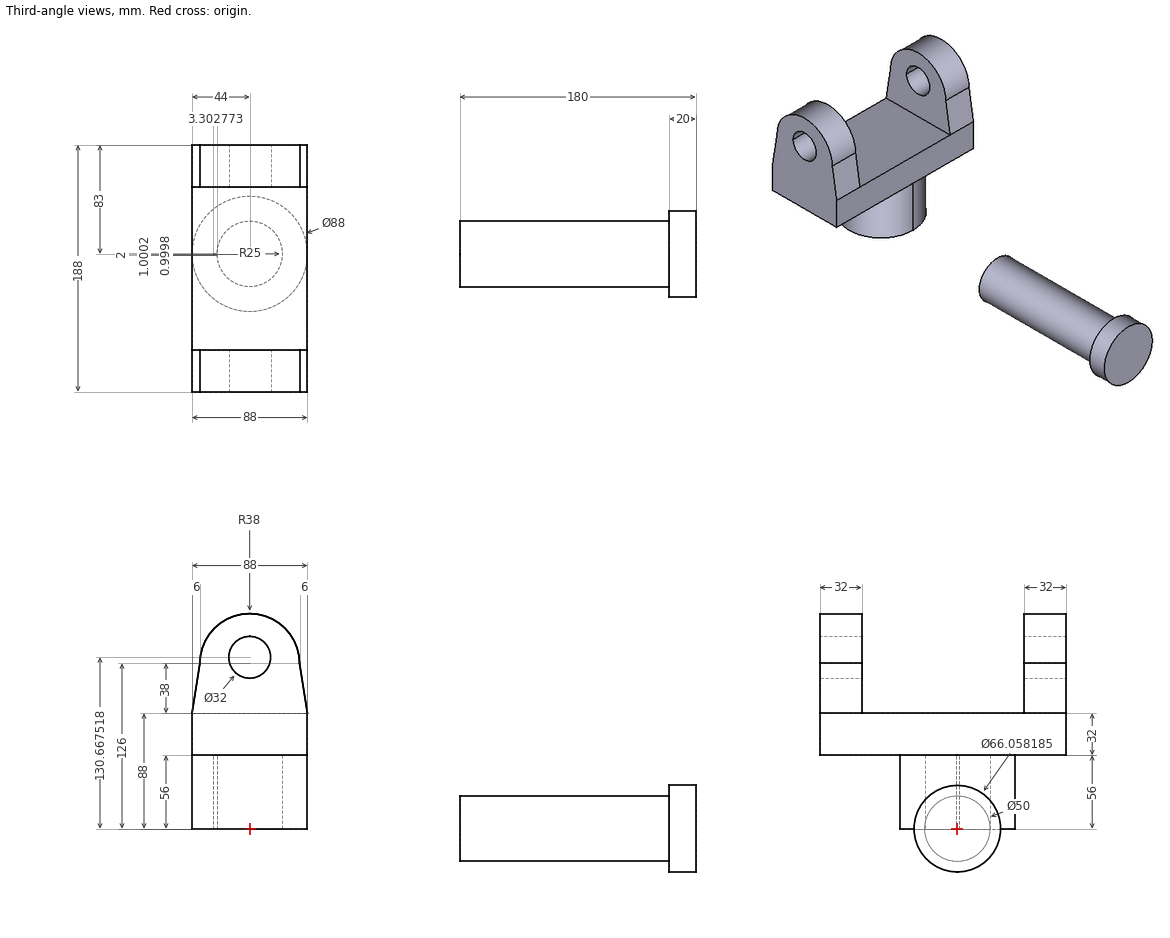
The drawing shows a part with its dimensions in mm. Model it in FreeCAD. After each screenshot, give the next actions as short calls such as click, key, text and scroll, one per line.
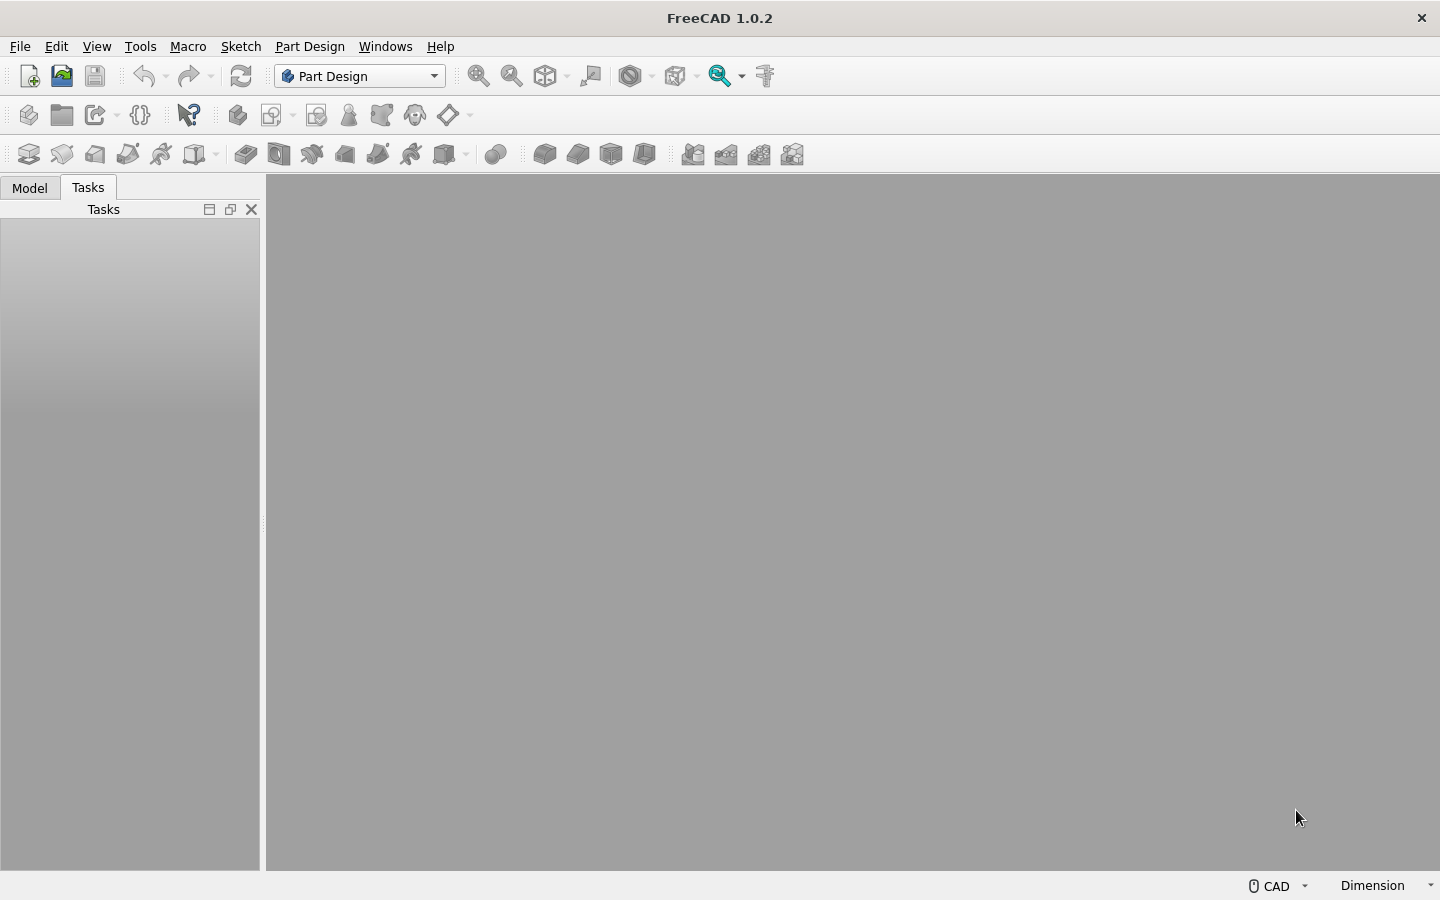
key(ctrl+n)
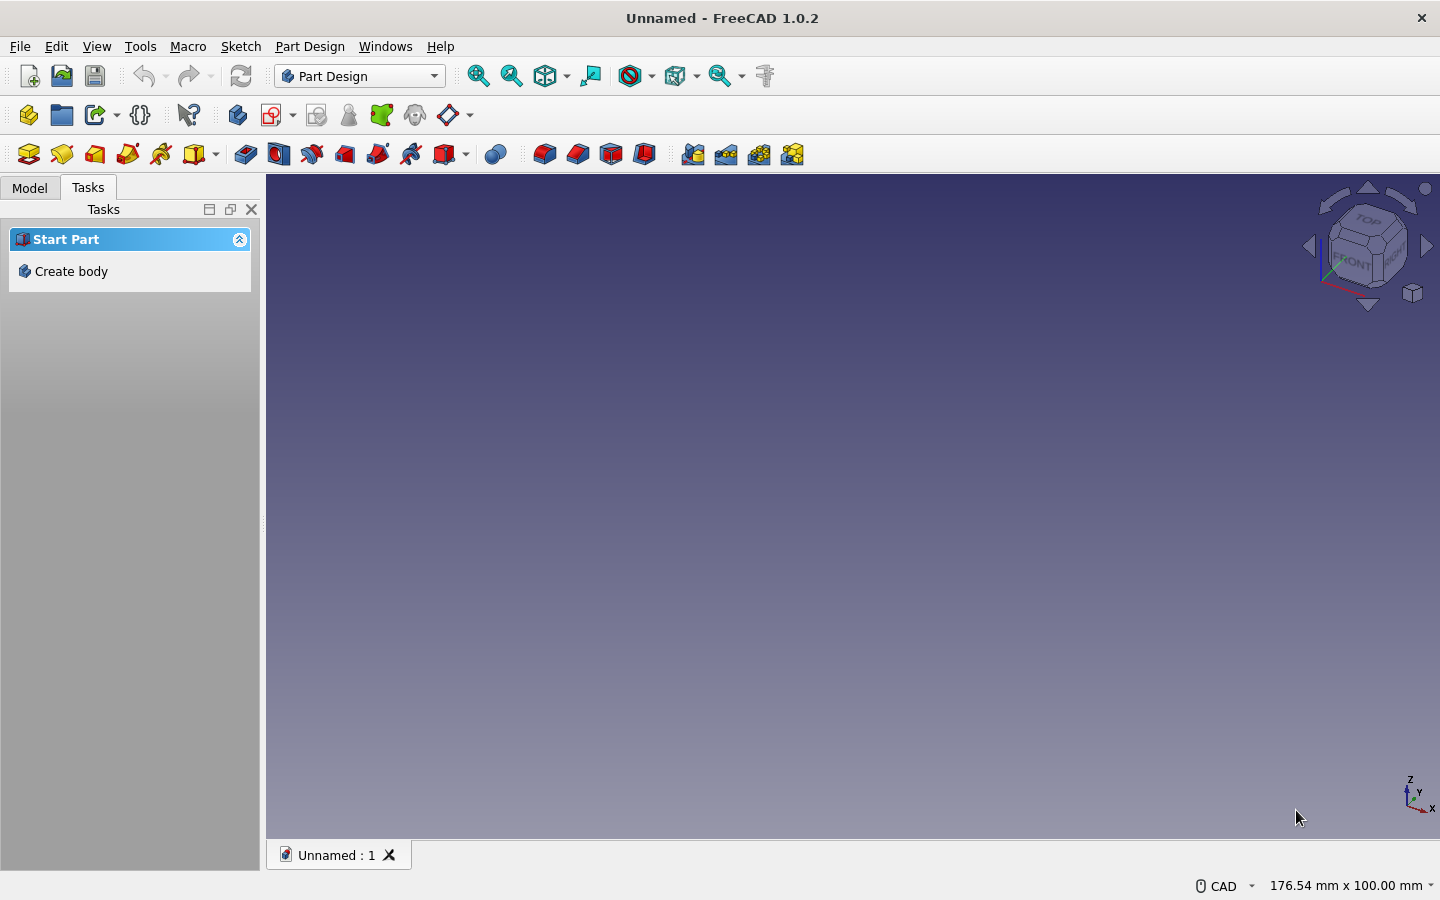
click(270, 116)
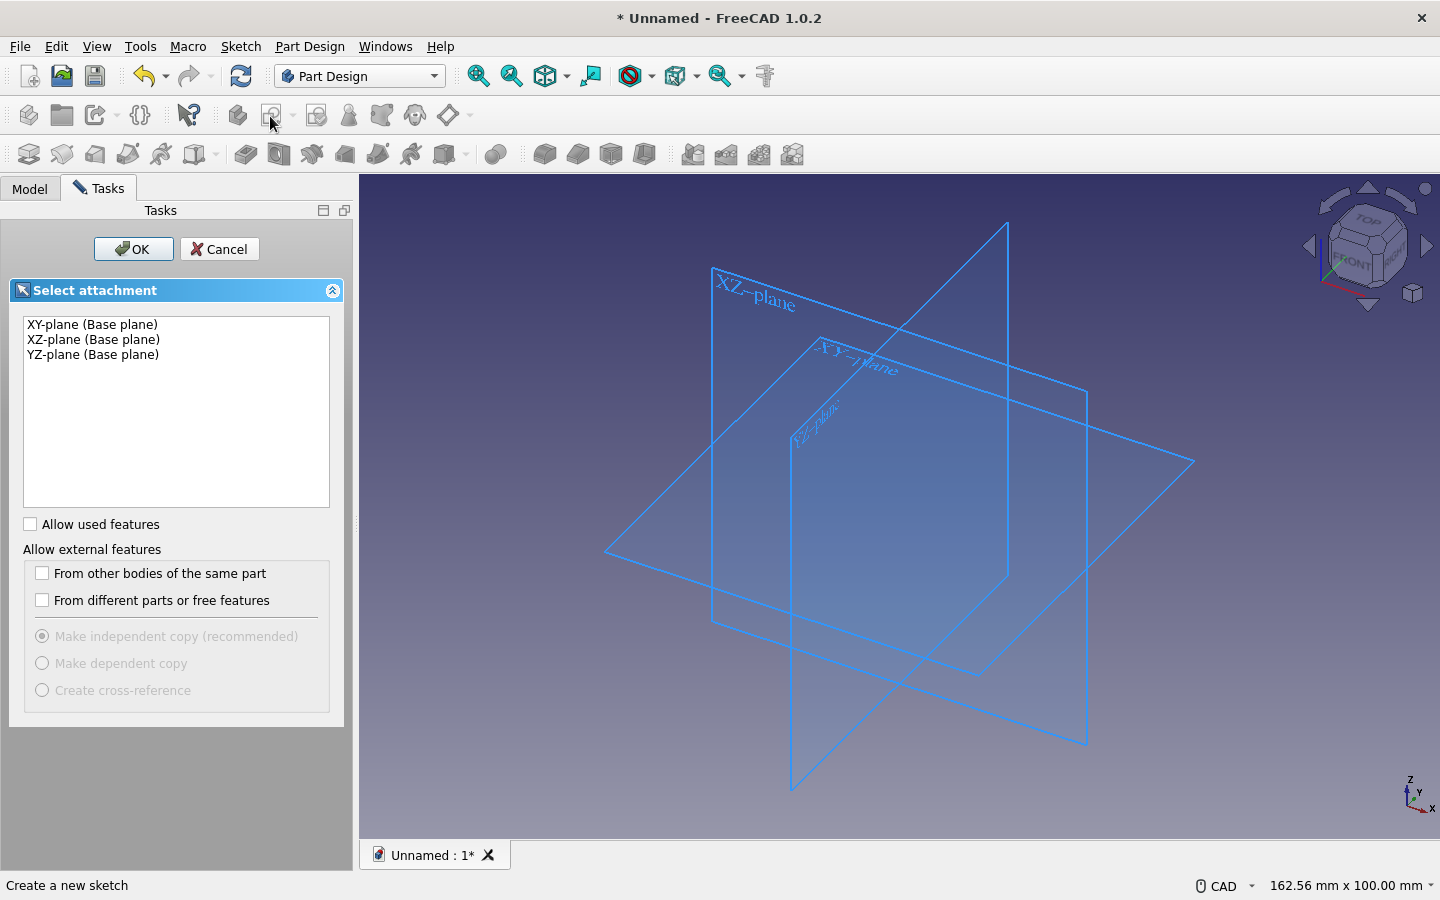
click(84, 324)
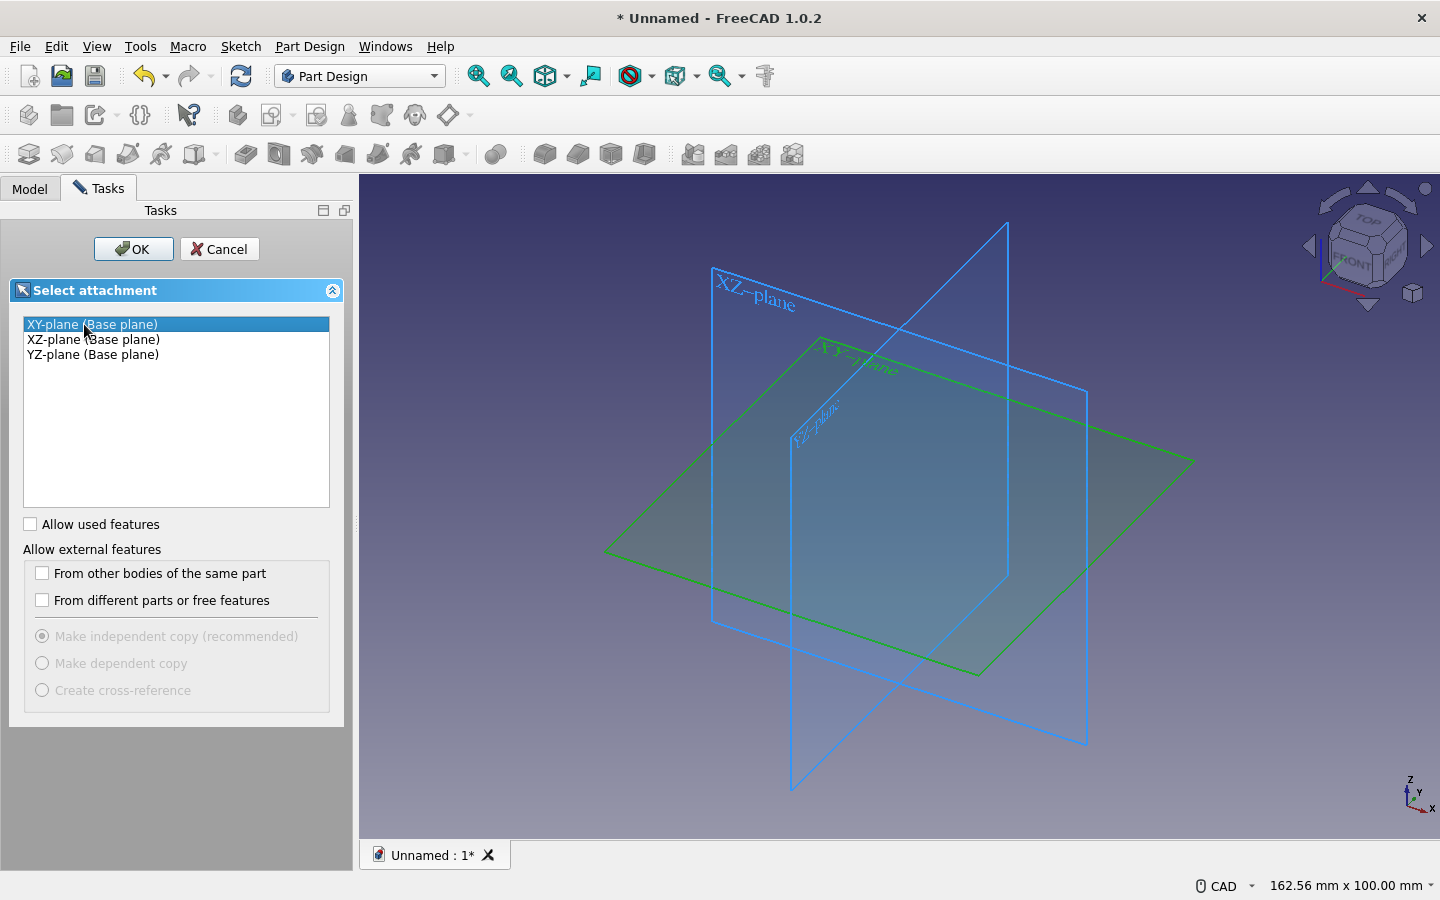
click(134, 249)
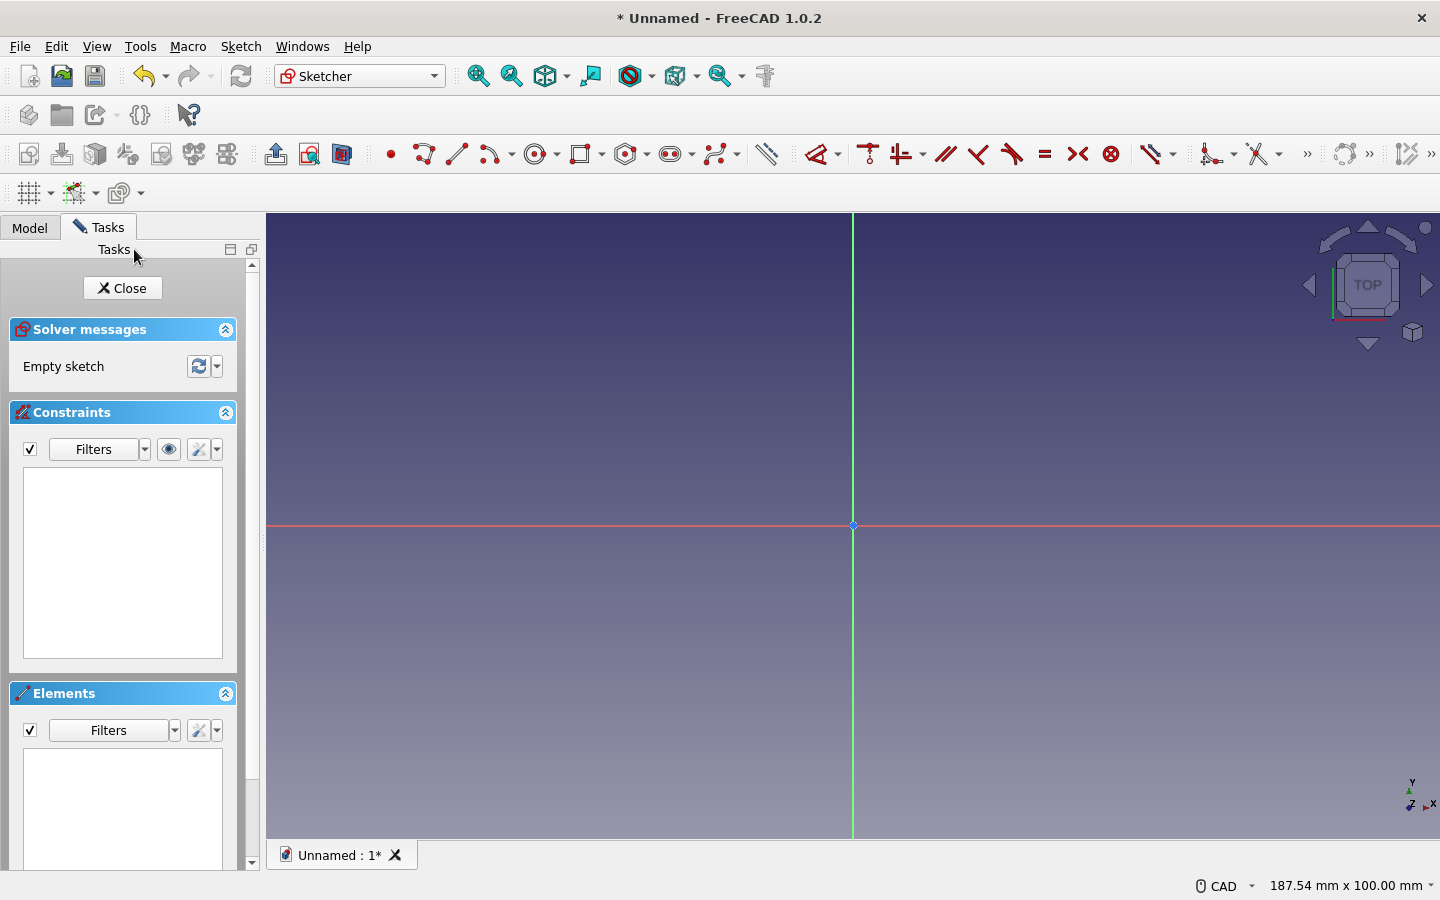
scroll(645, 526, down, 2)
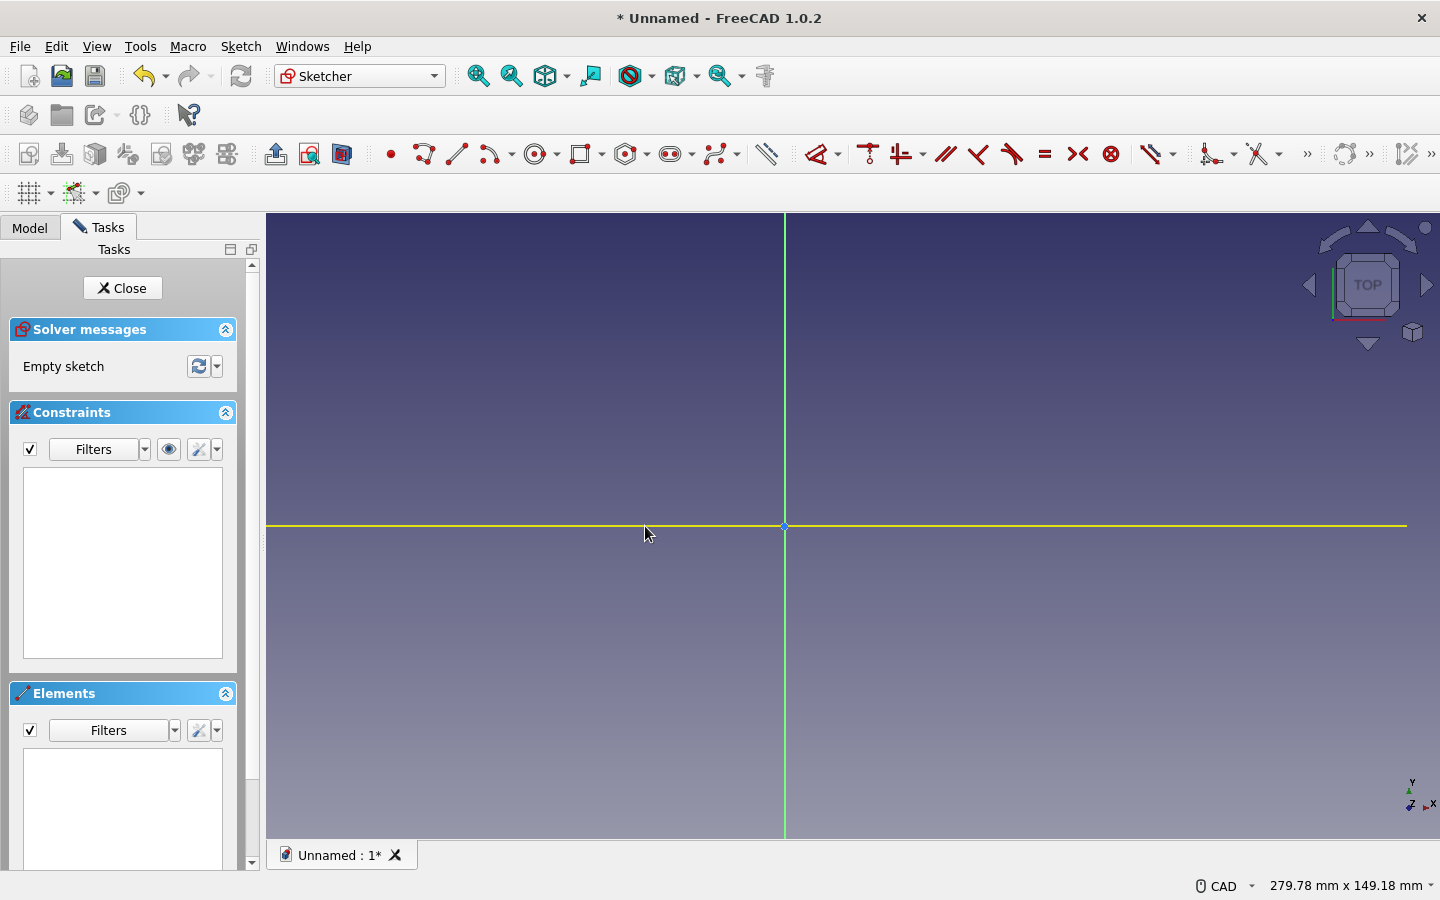
key(g)
key(c)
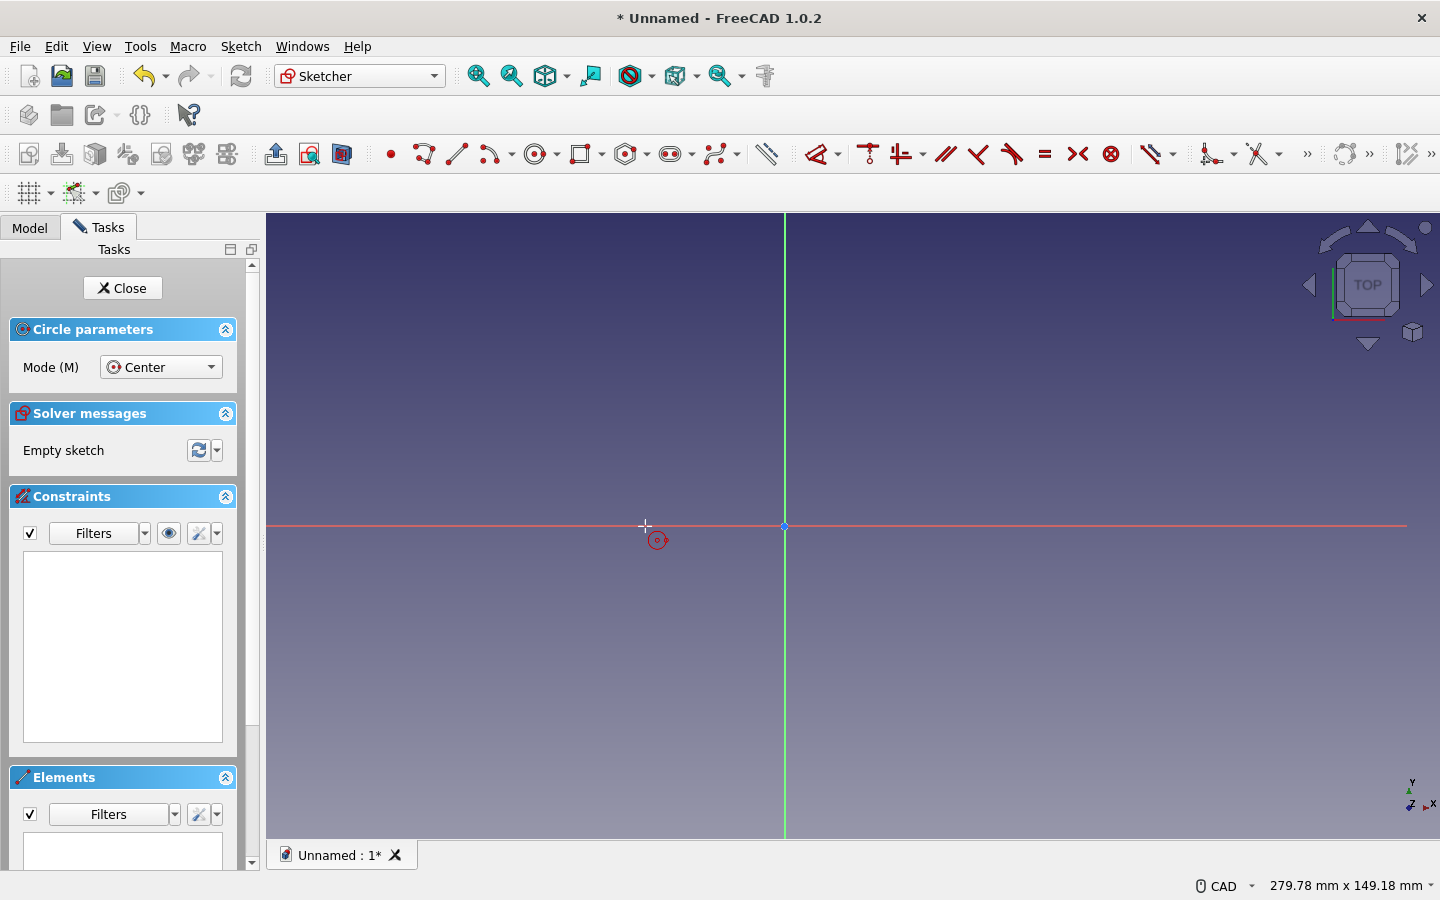
click(785, 526)
click(915, 396)
key(Escape)